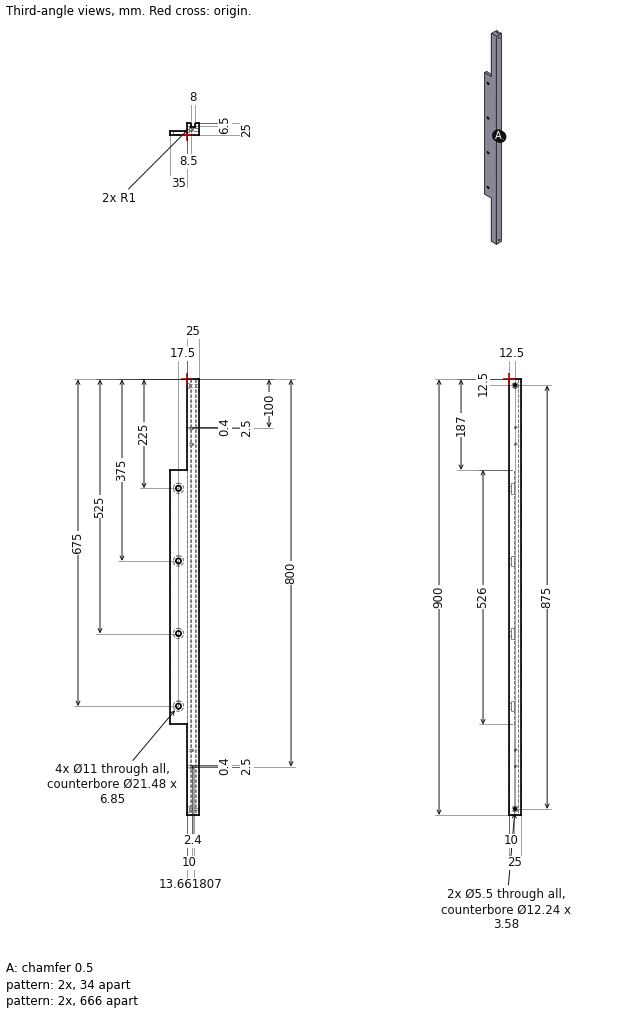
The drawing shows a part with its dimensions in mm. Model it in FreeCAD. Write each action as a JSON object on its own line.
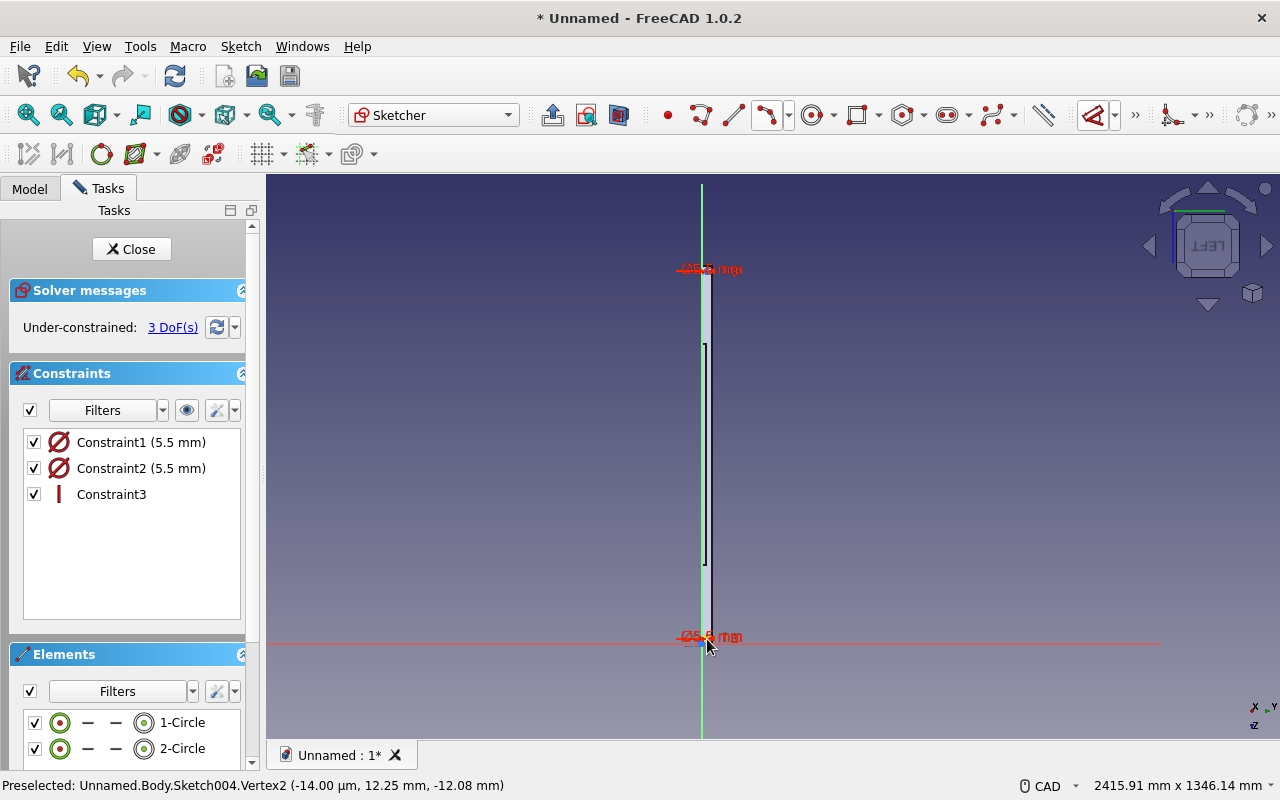
{"action": "scroll", "coordinate": [707, 271], "scroll_direction": "up", "scroll_amount": 11}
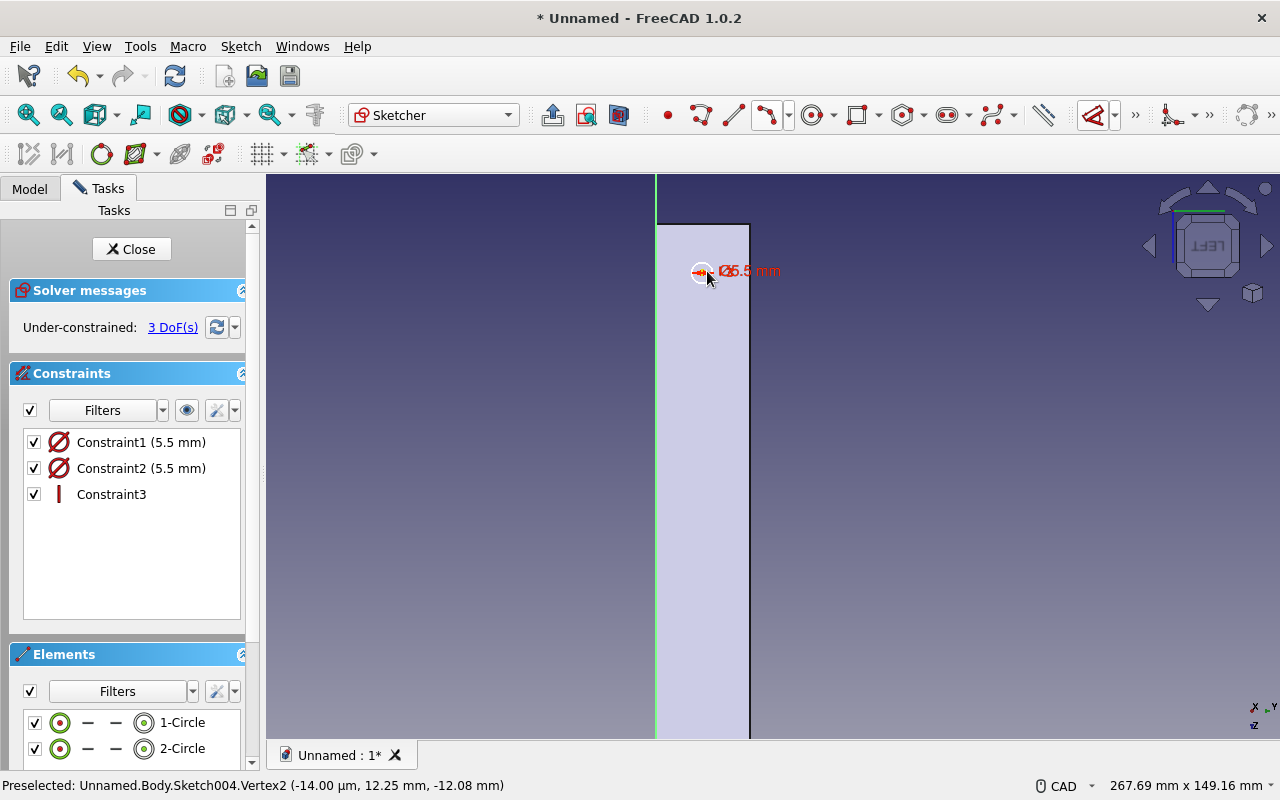
{"action": "left_click", "coordinate": [702, 273]}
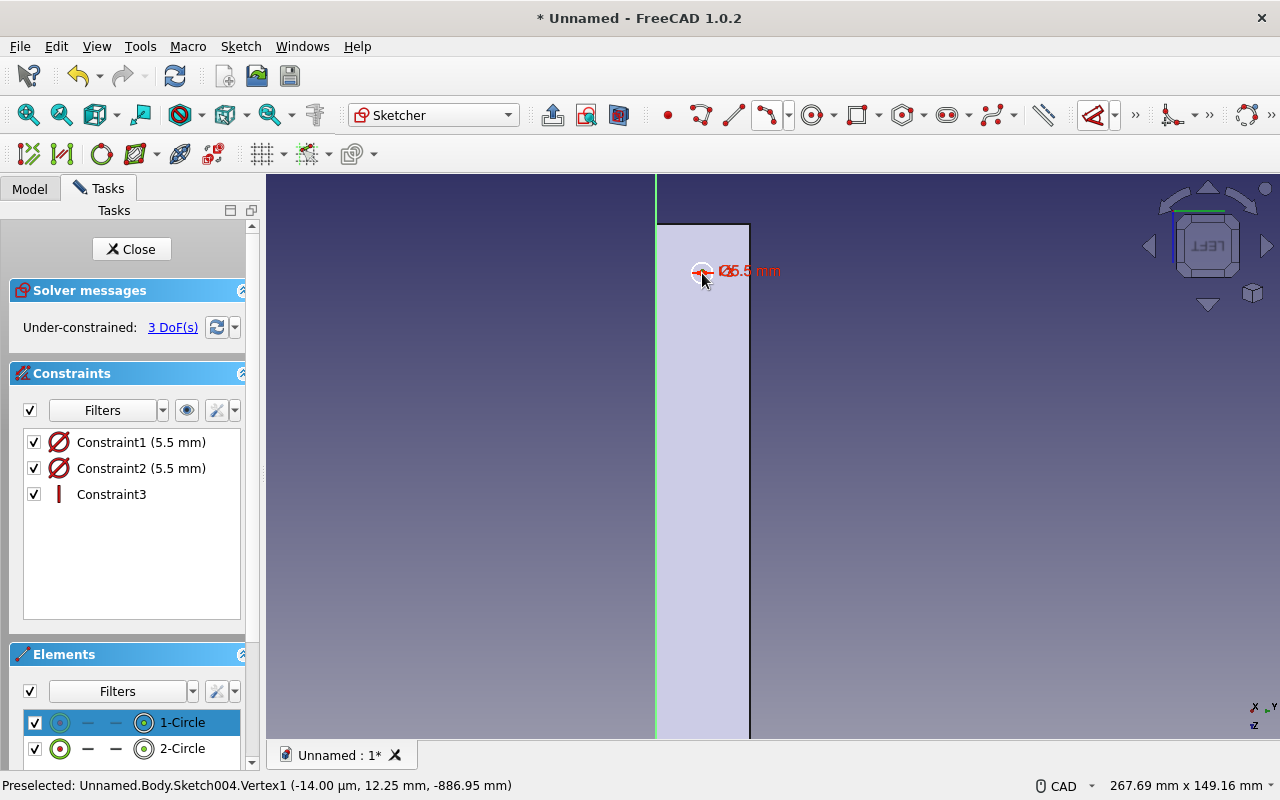
{"action": "key", "text": "l"}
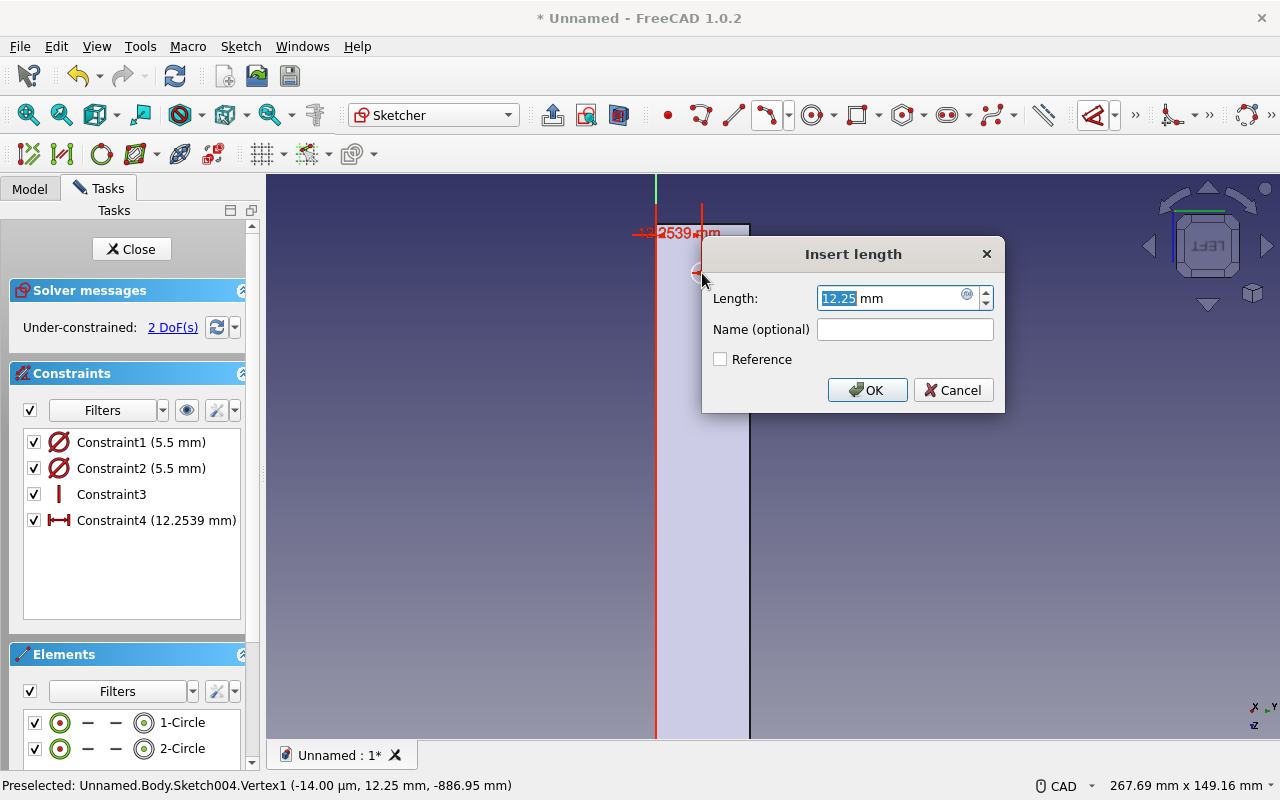
{"action": "type", "text": "12.5"}
{"action": "key", "text": "Return"}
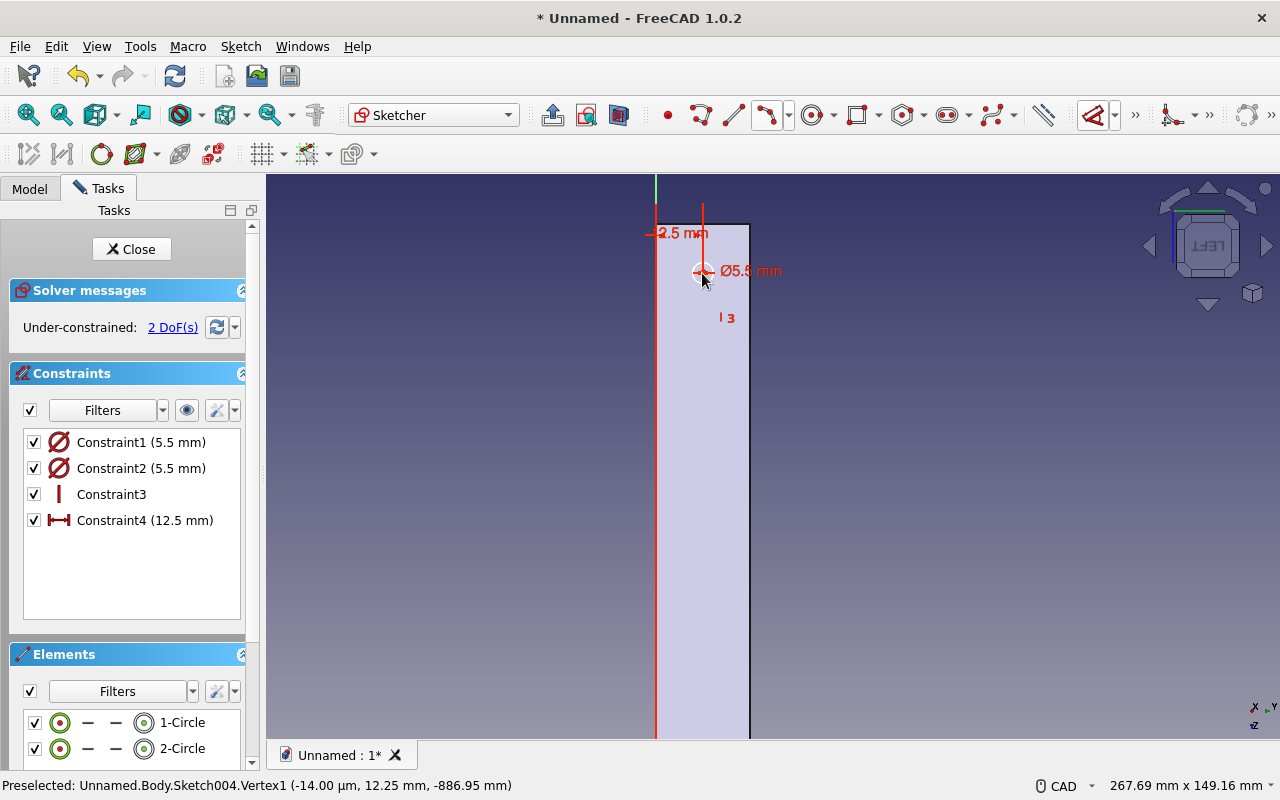
{"action": "scroll", "coordinate": [707, 271], "scroll_direction": "down", "scroll_amount": 11}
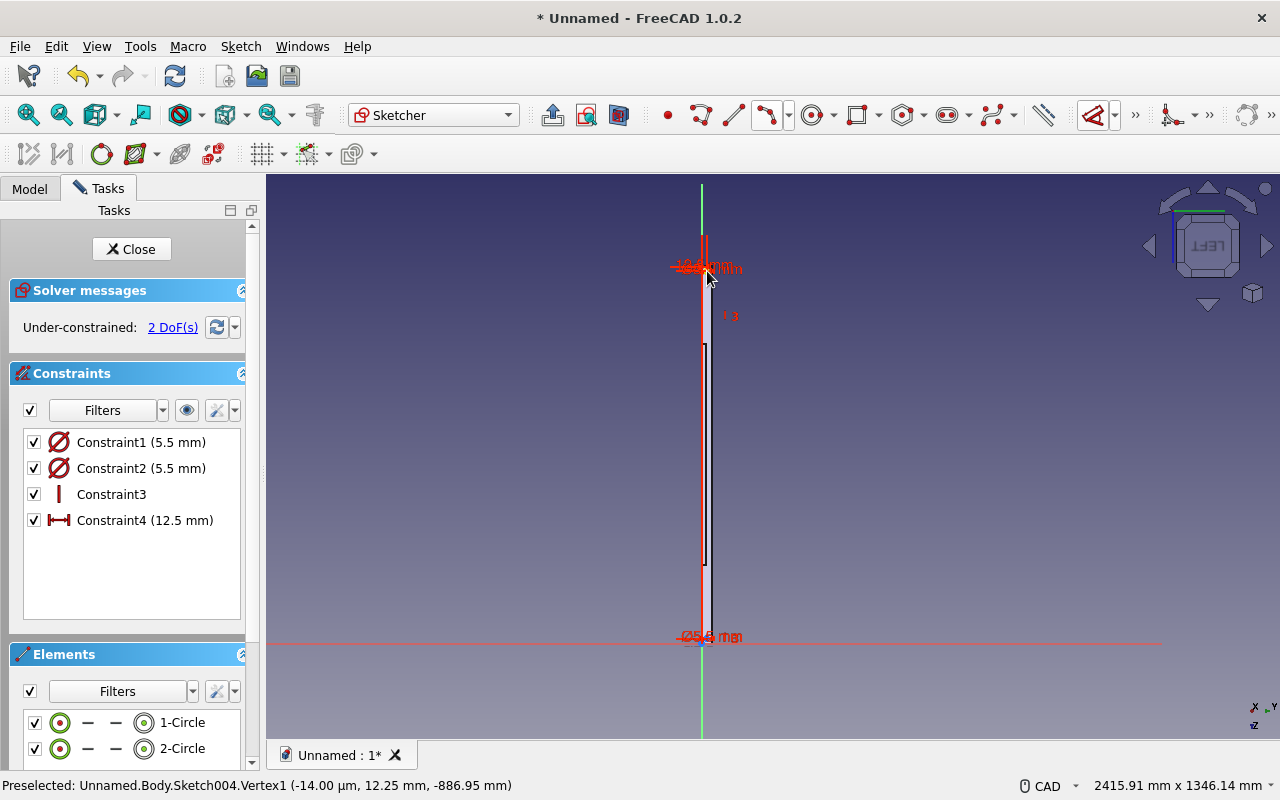
{"action": "scroll", "coordinate": [707, 639], "scroll_direction": "up", "scroll_amount": 11}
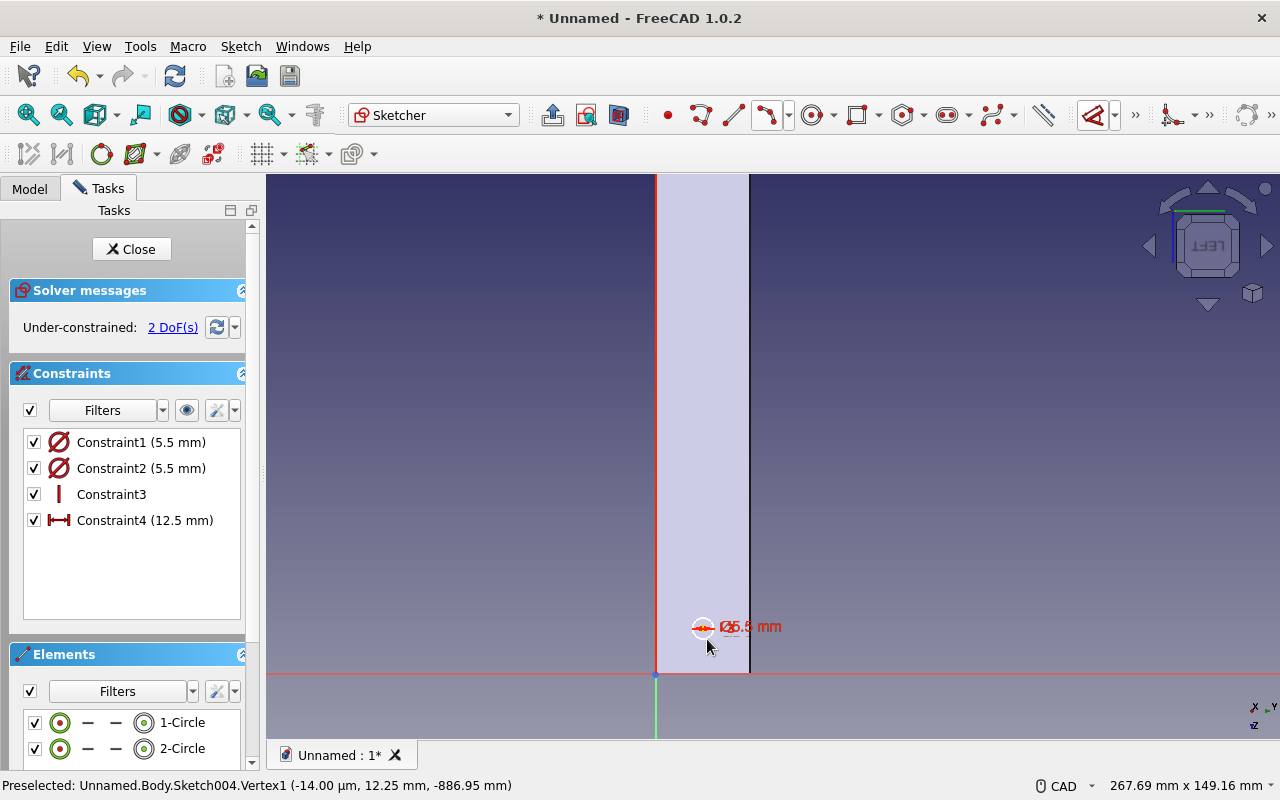
{"action": "left_click", "coordinate": [703, 629]}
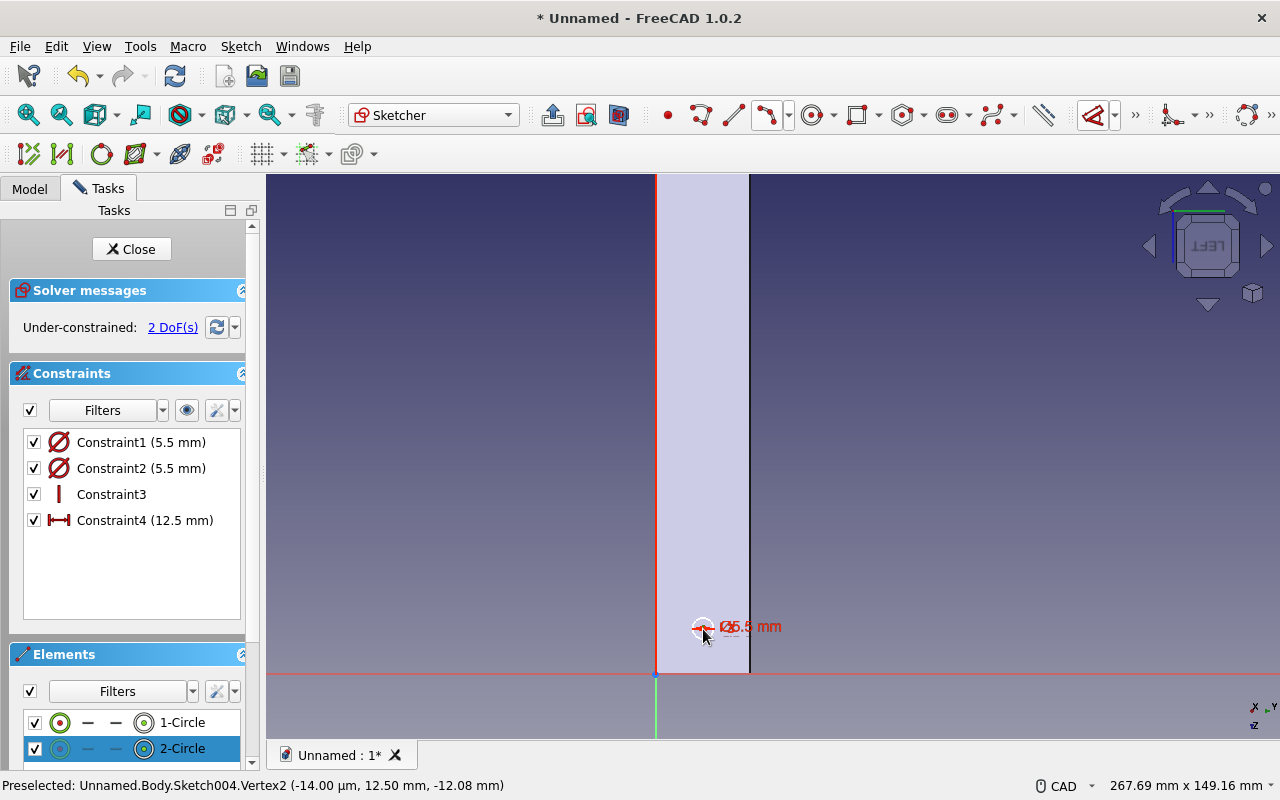
{"action": "key", "text": "i"}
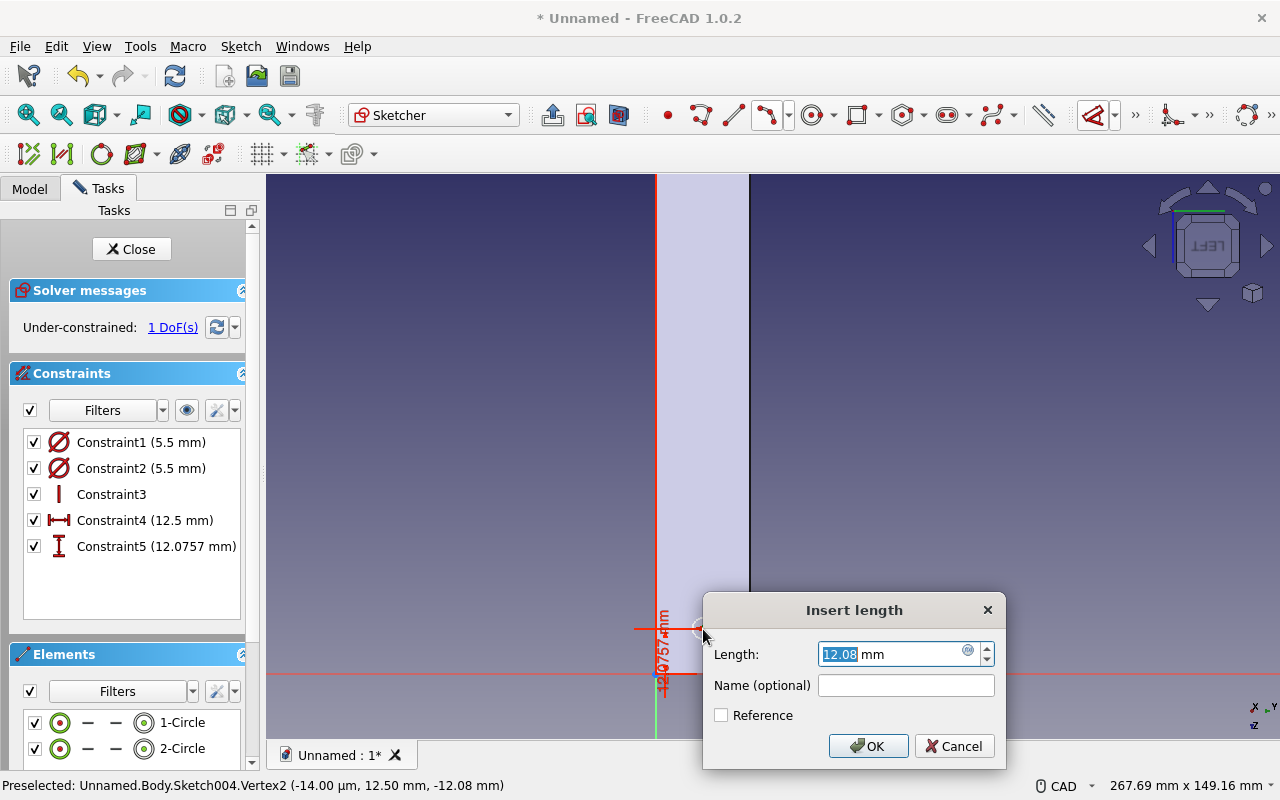
{"action": "type", "text": "12.5"}
{"action": "key", "text": "Return"}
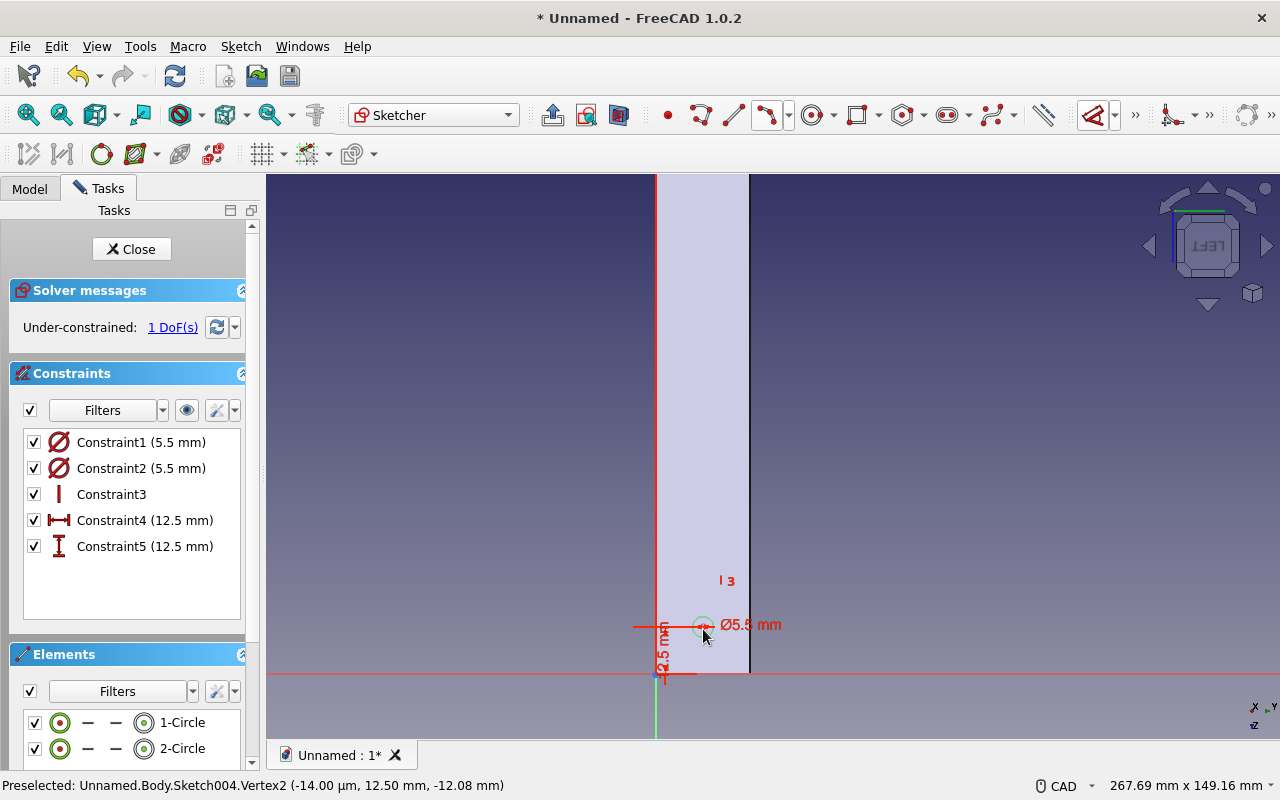
{"action": "scroll", "coordinate": [707, 639], "scroll_direction": "down", "scroll_amount": 11}